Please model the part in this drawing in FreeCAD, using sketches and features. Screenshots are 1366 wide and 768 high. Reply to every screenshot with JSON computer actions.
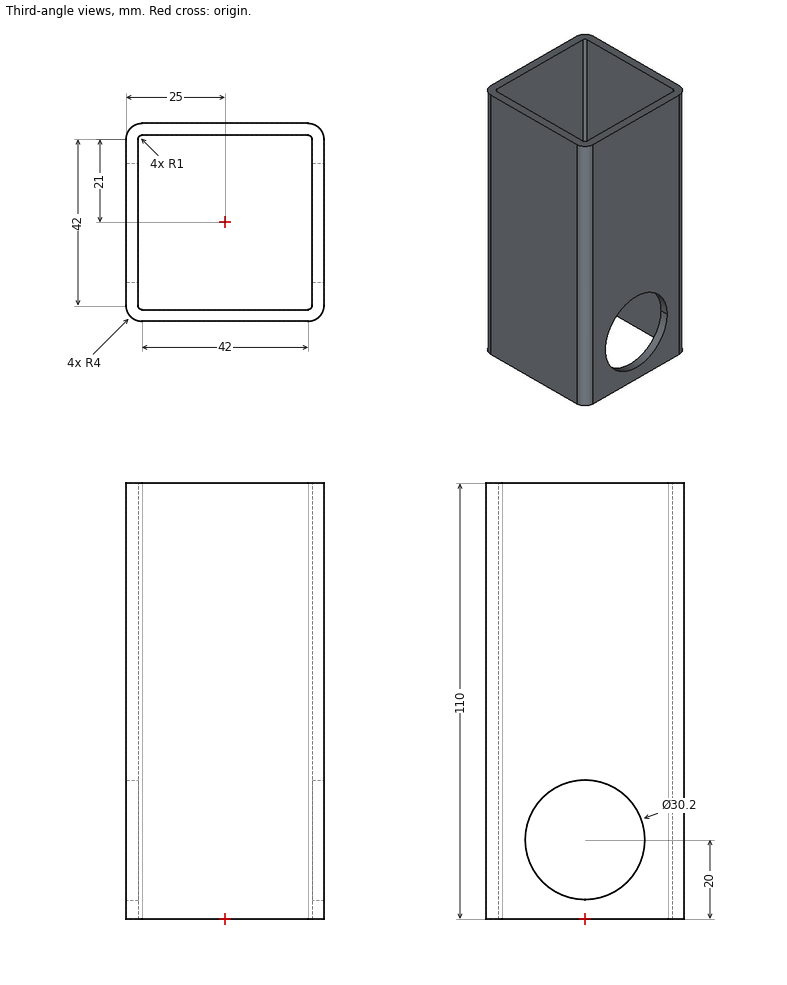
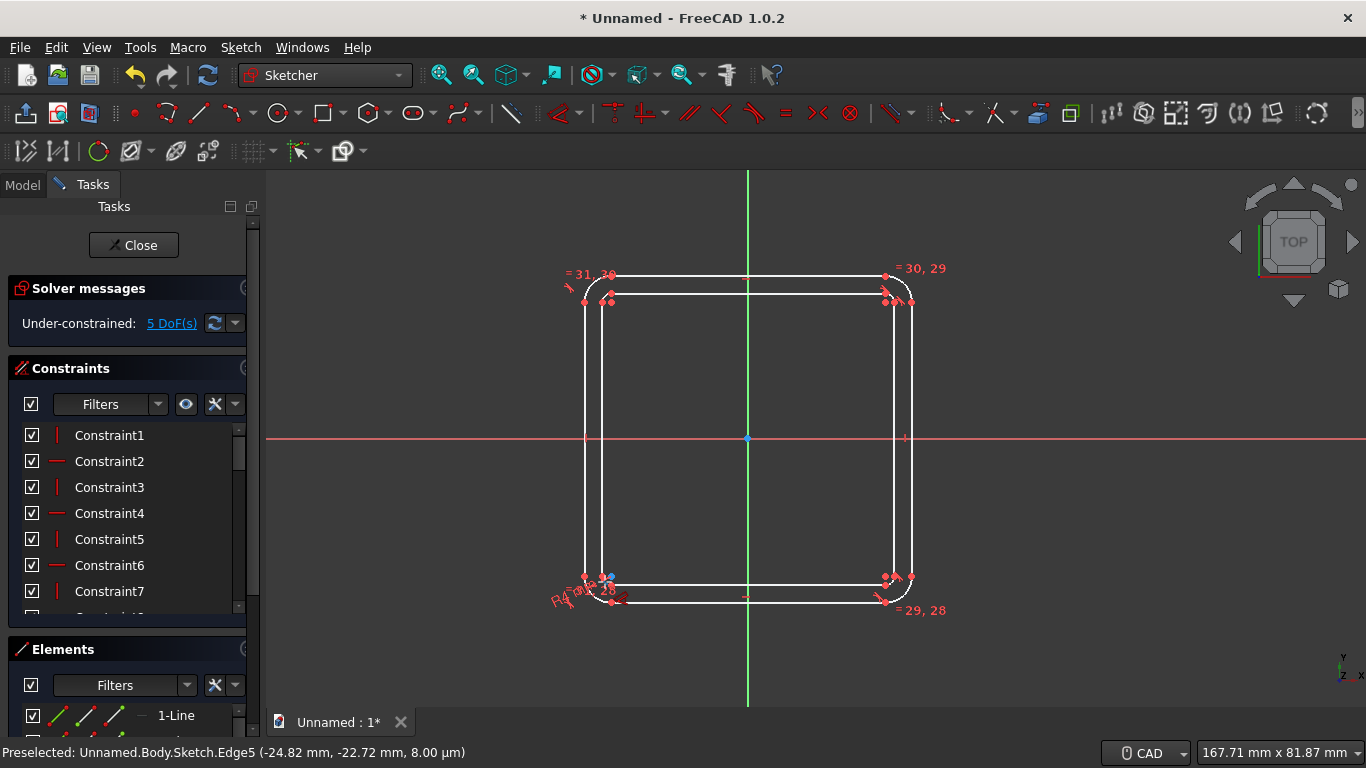
{"action": "scroll", "coordinate": [607, 295], "scroll_direction": "up", "scroll_amount": 10}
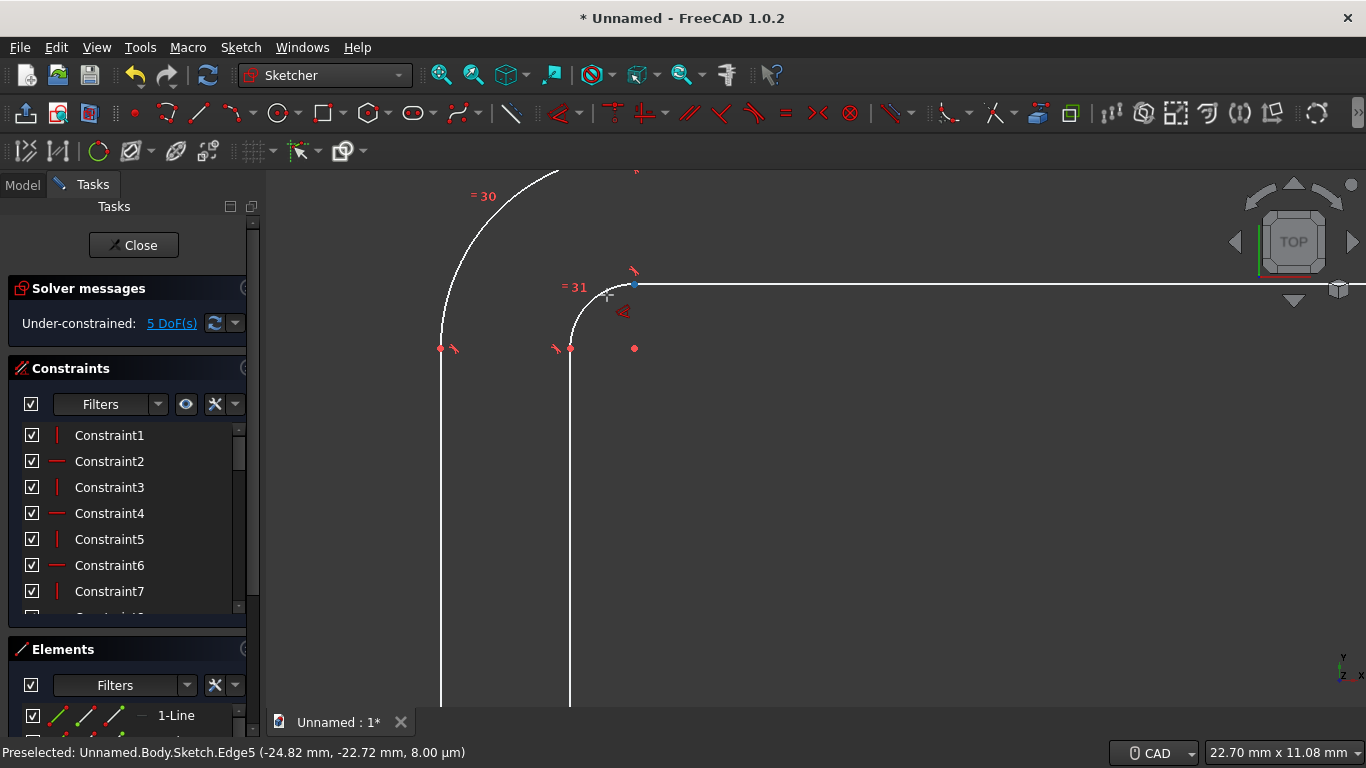
{"action": "left_click", "coordinate": [605, 291]}
{"action": "left_click", "coordinate": [590, 263]}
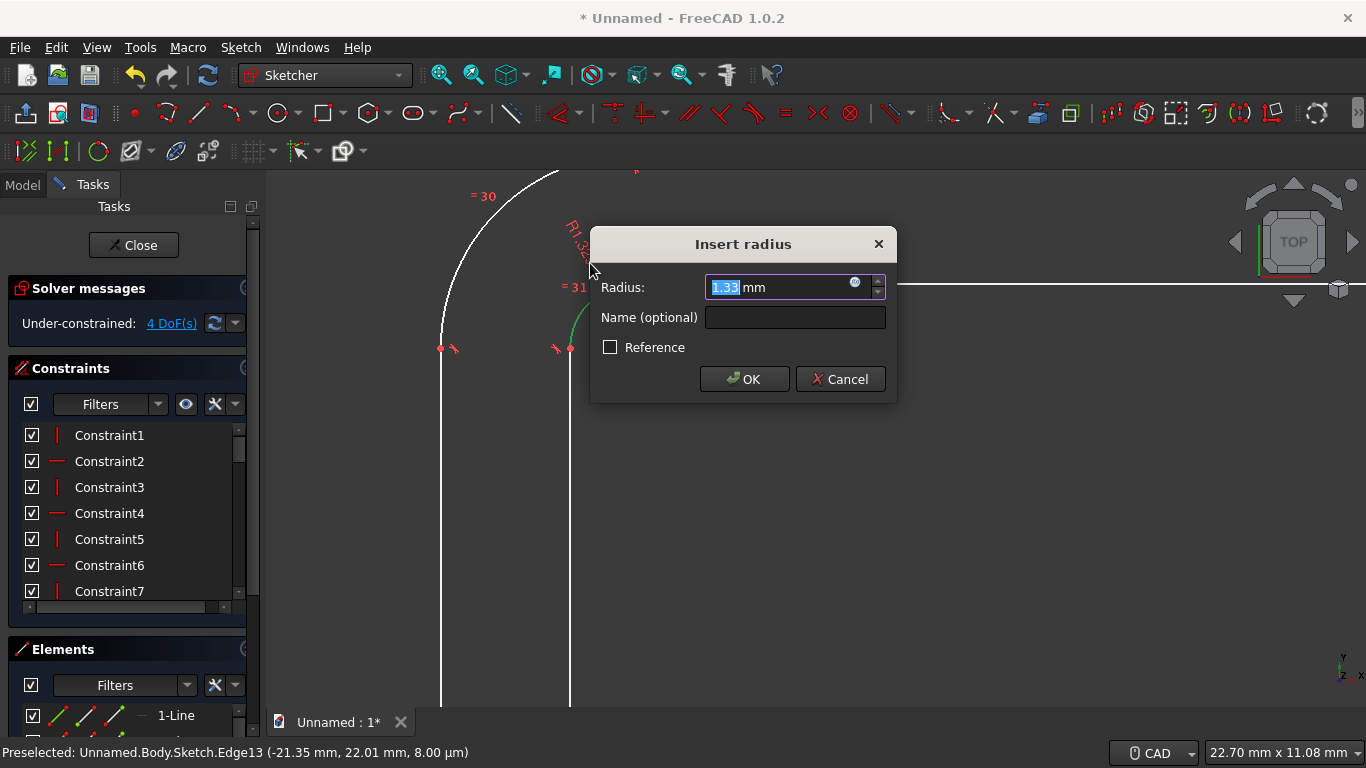
{"action": "type", "text": "1"}
{"action": "key", "text": "Return"}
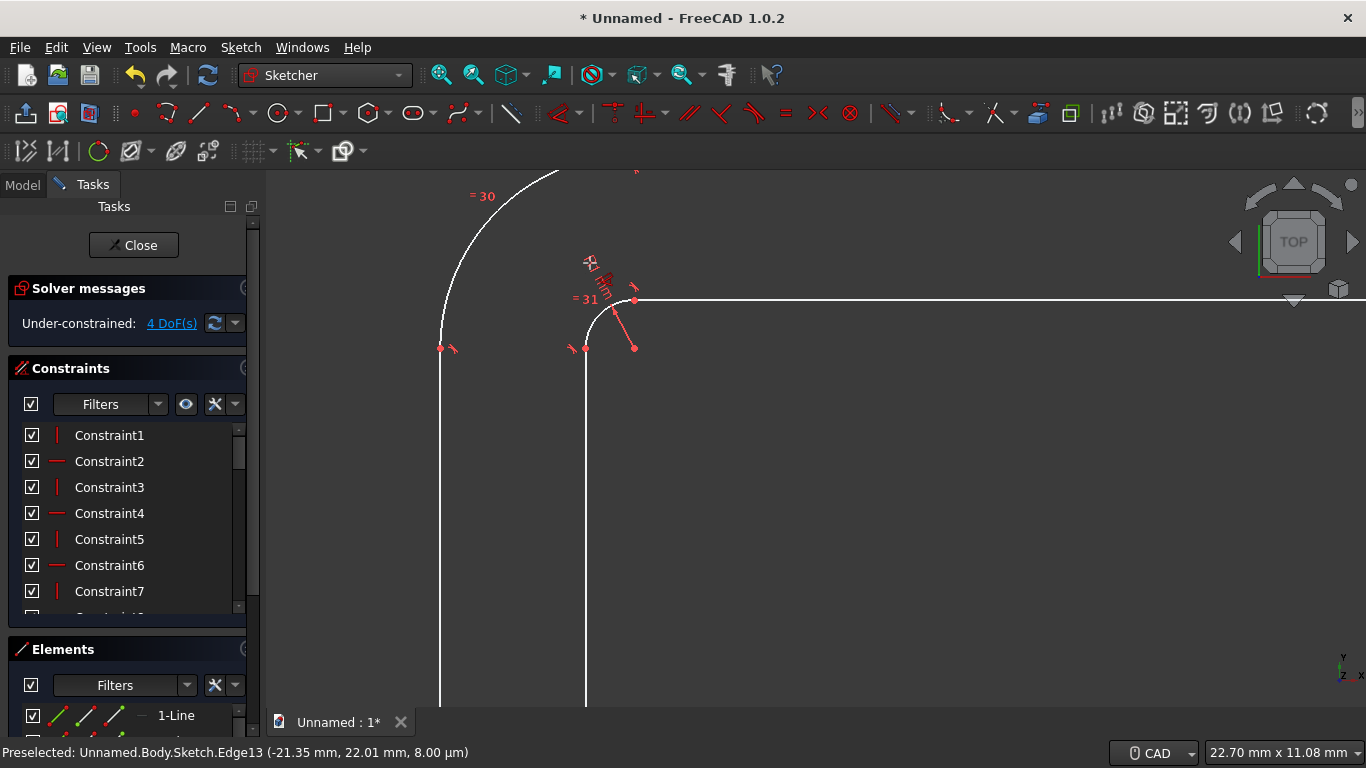
{"action": "scroll", "coordinate": [607, 295], "scroll_direction": "down", "scroll_amount": 10}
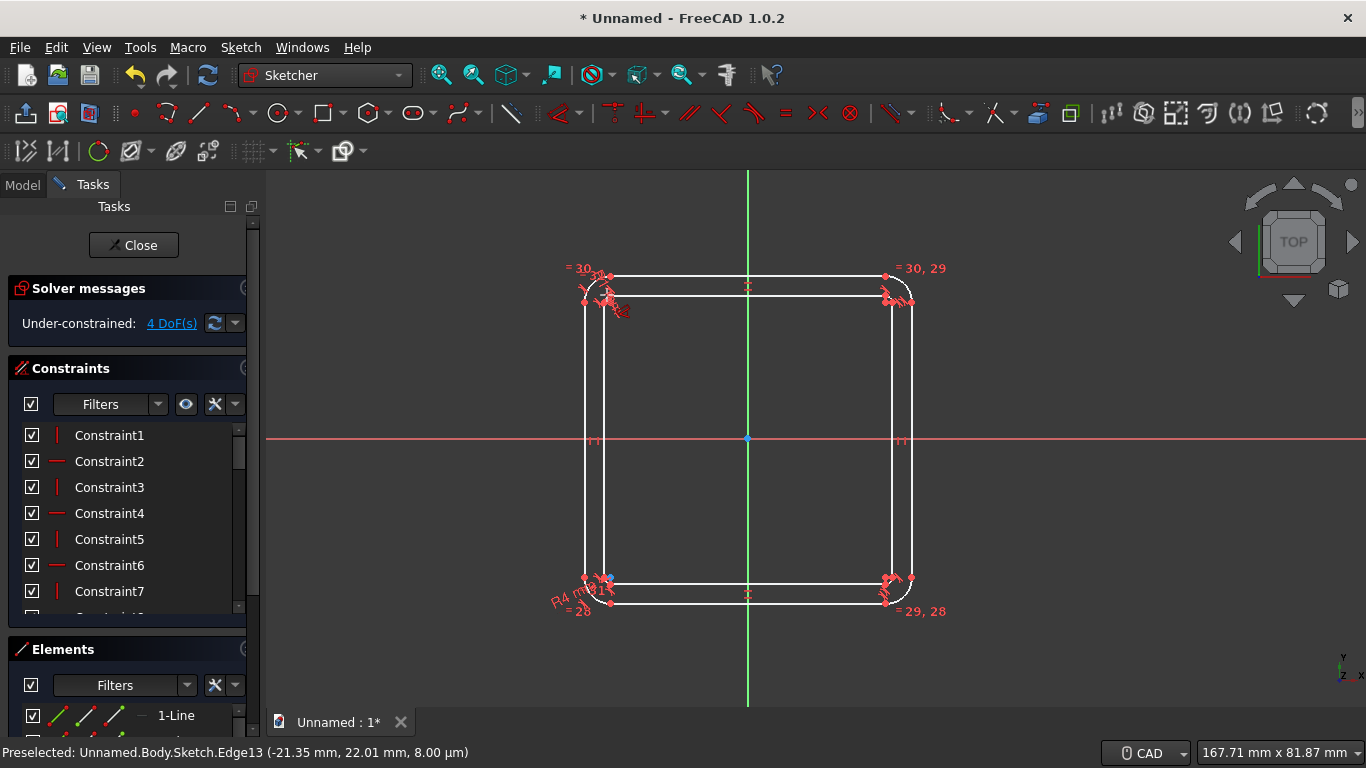
{"action": "left_click", "coordinate": [585, 385]}
{"action": "left_click", "coordinate": [551, 377]}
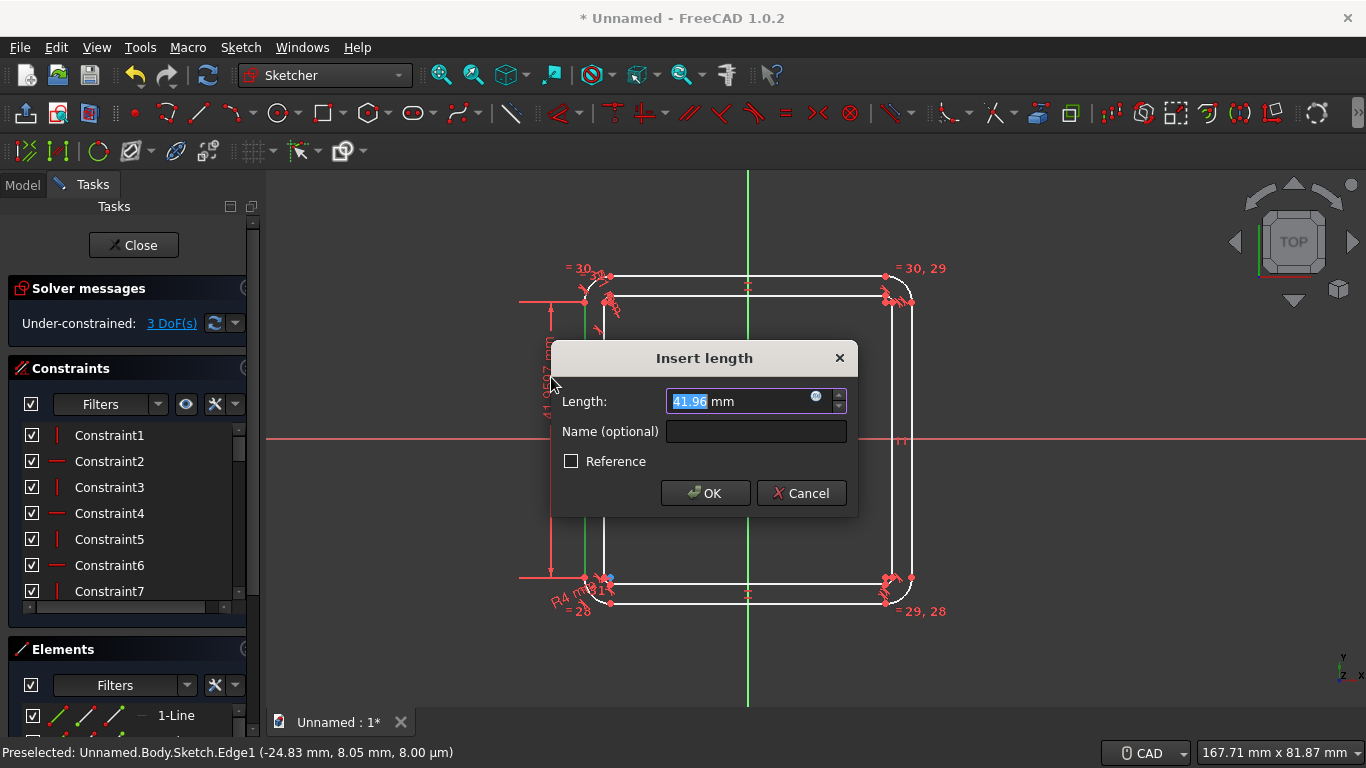
{"action": "type", "text": "42"}
{"action": "key", "text": "Return"}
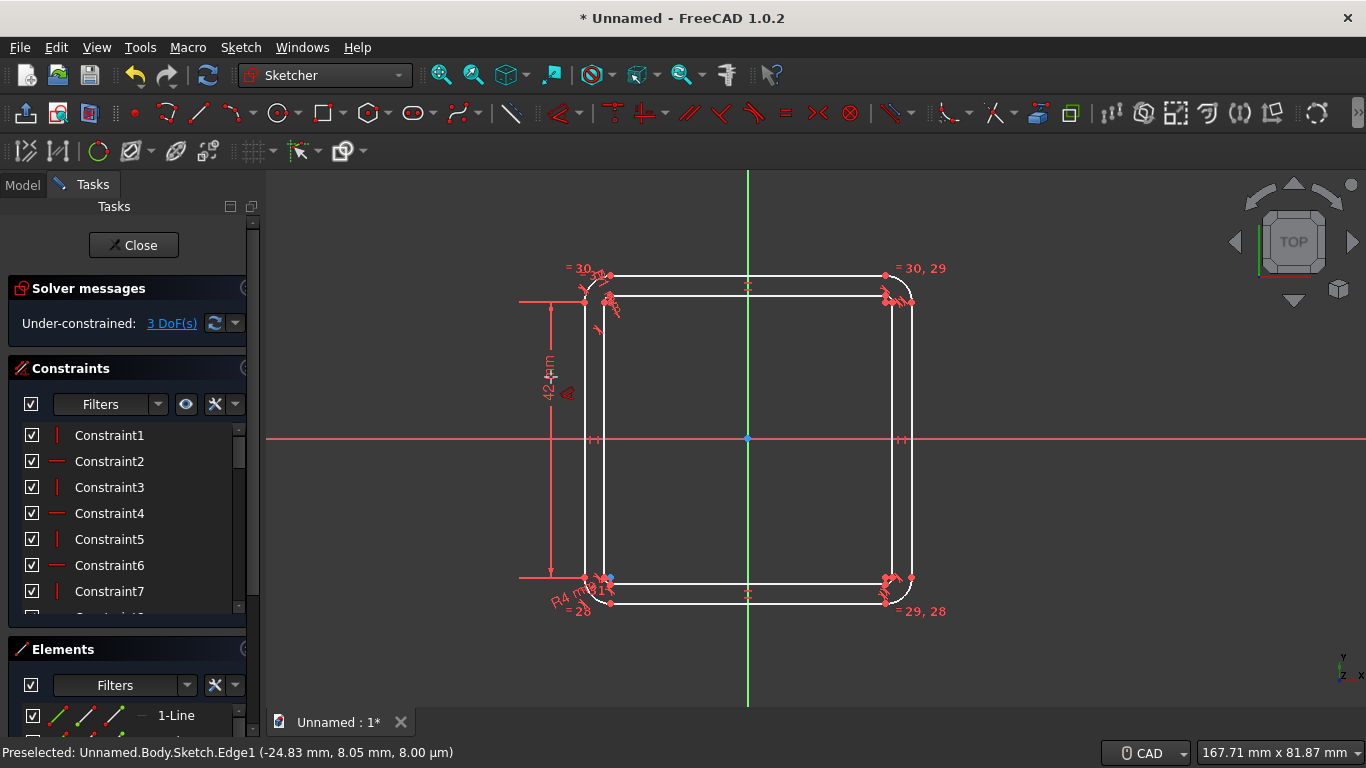
{"action": "left_click", "coordinate": [693, 604]}
{"action": "left_click", "coordinate": [685, 638]}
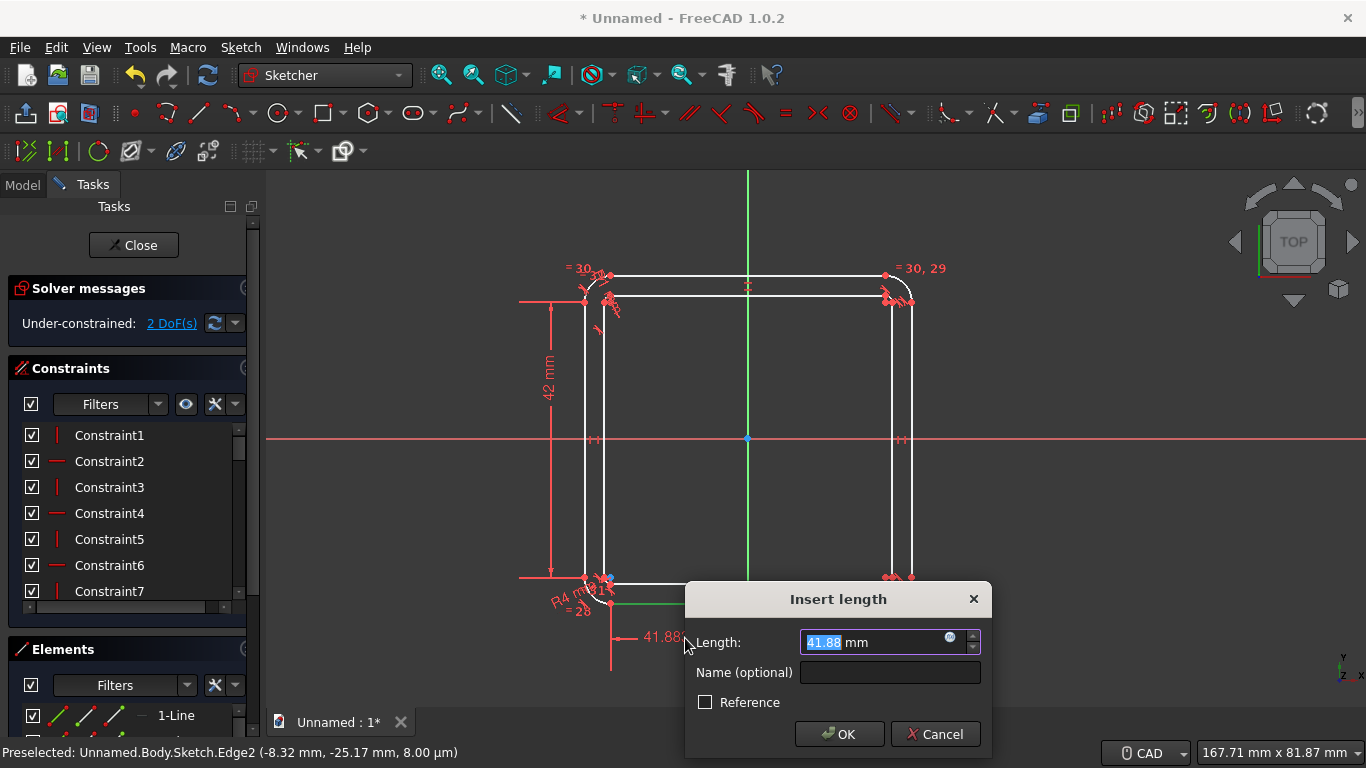
{"action": "type", "text": "42"}
{"action": "key", "text": "Return"}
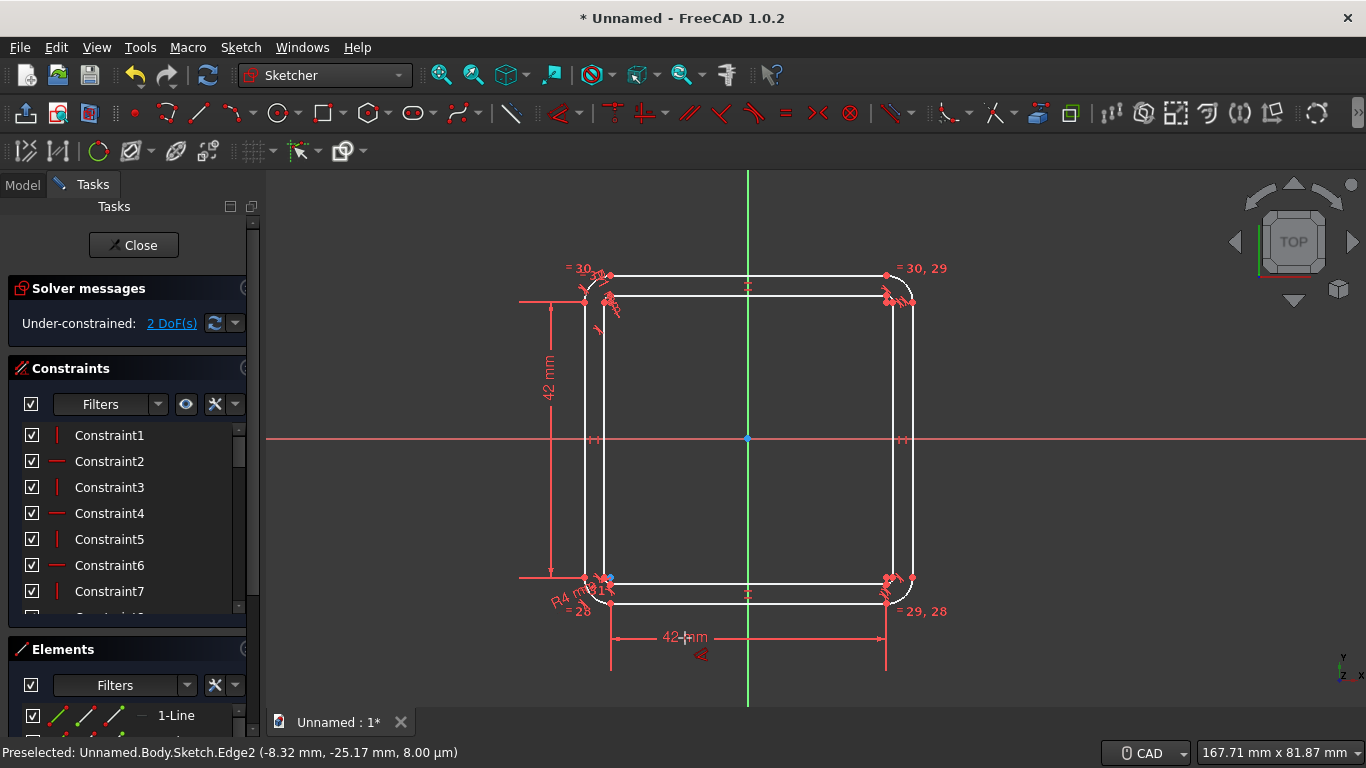
{"action": "left_click", "coordinate": [585, 302]}
{"action": "left_click", "coordinate": [666, 473]}